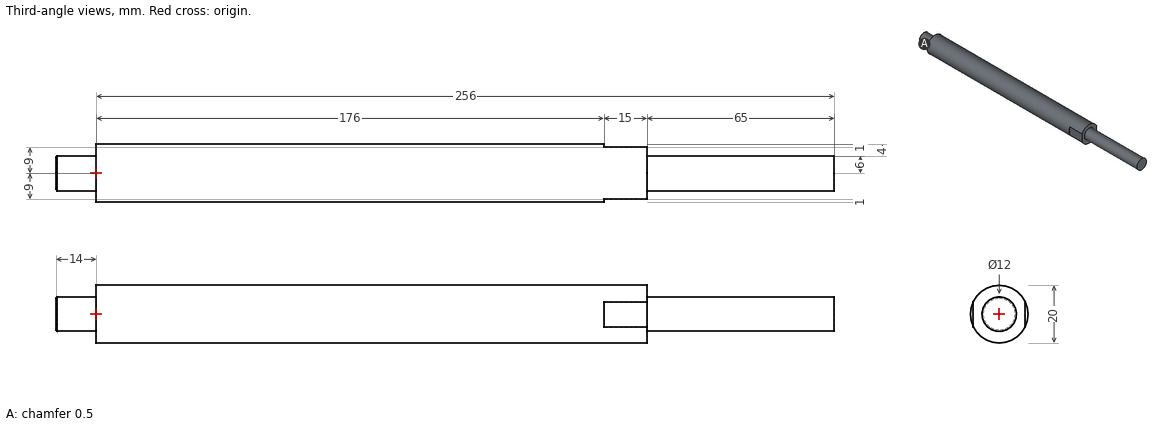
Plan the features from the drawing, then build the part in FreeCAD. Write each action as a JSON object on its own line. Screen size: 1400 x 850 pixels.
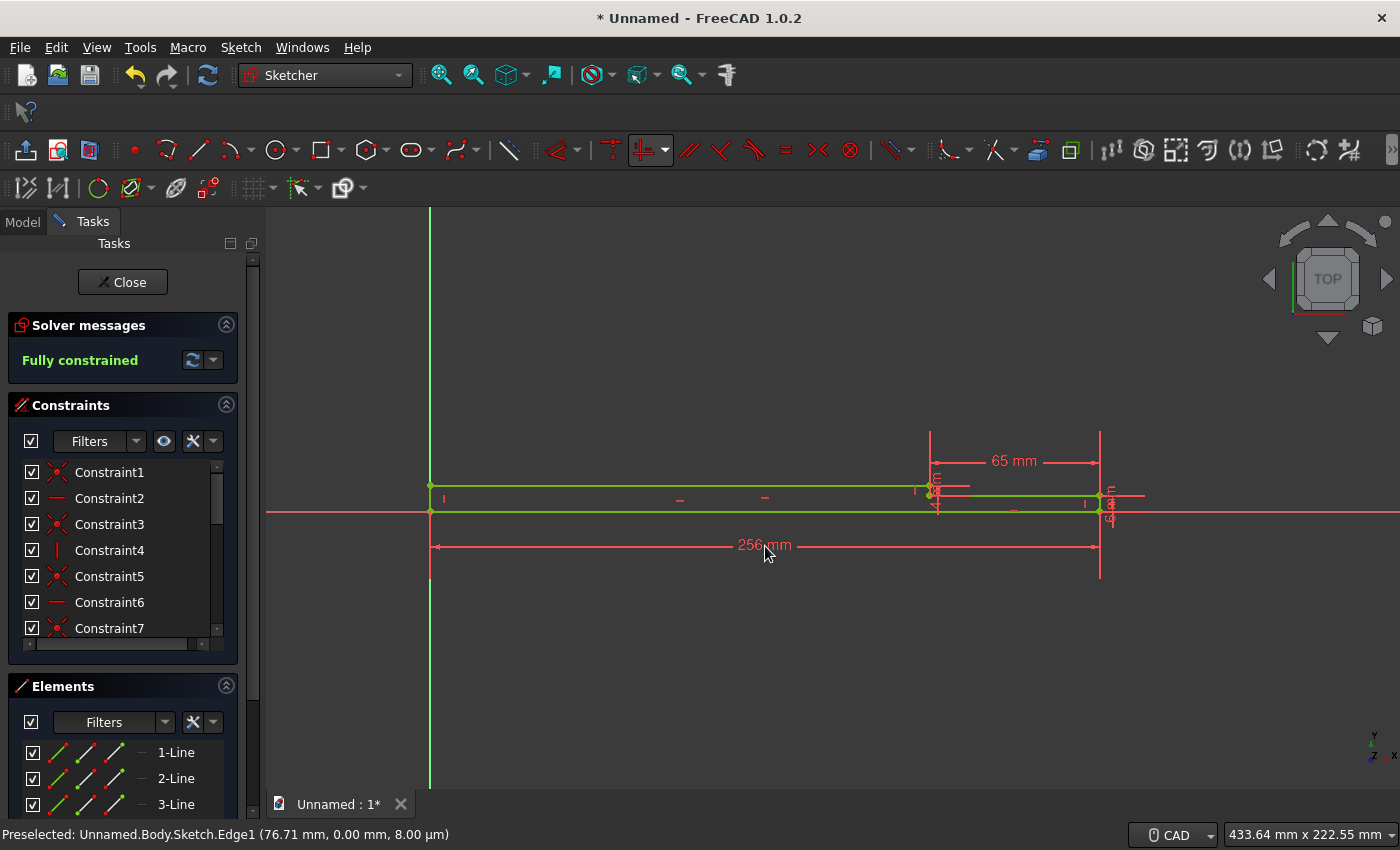
{"action": "left_click", "coordinate": [123, 282]}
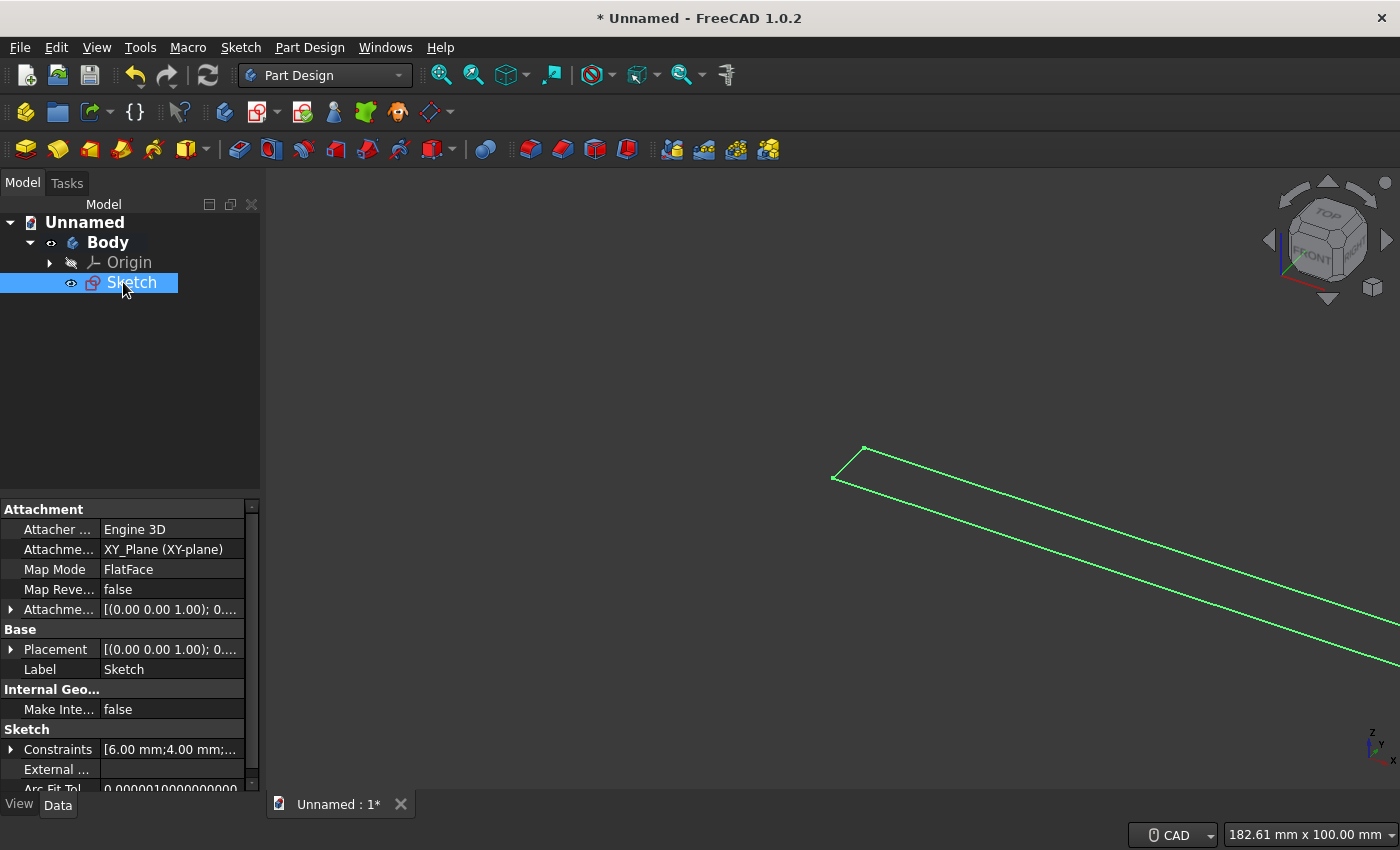
{"action": "left_click", "coordinate": [58, 150]}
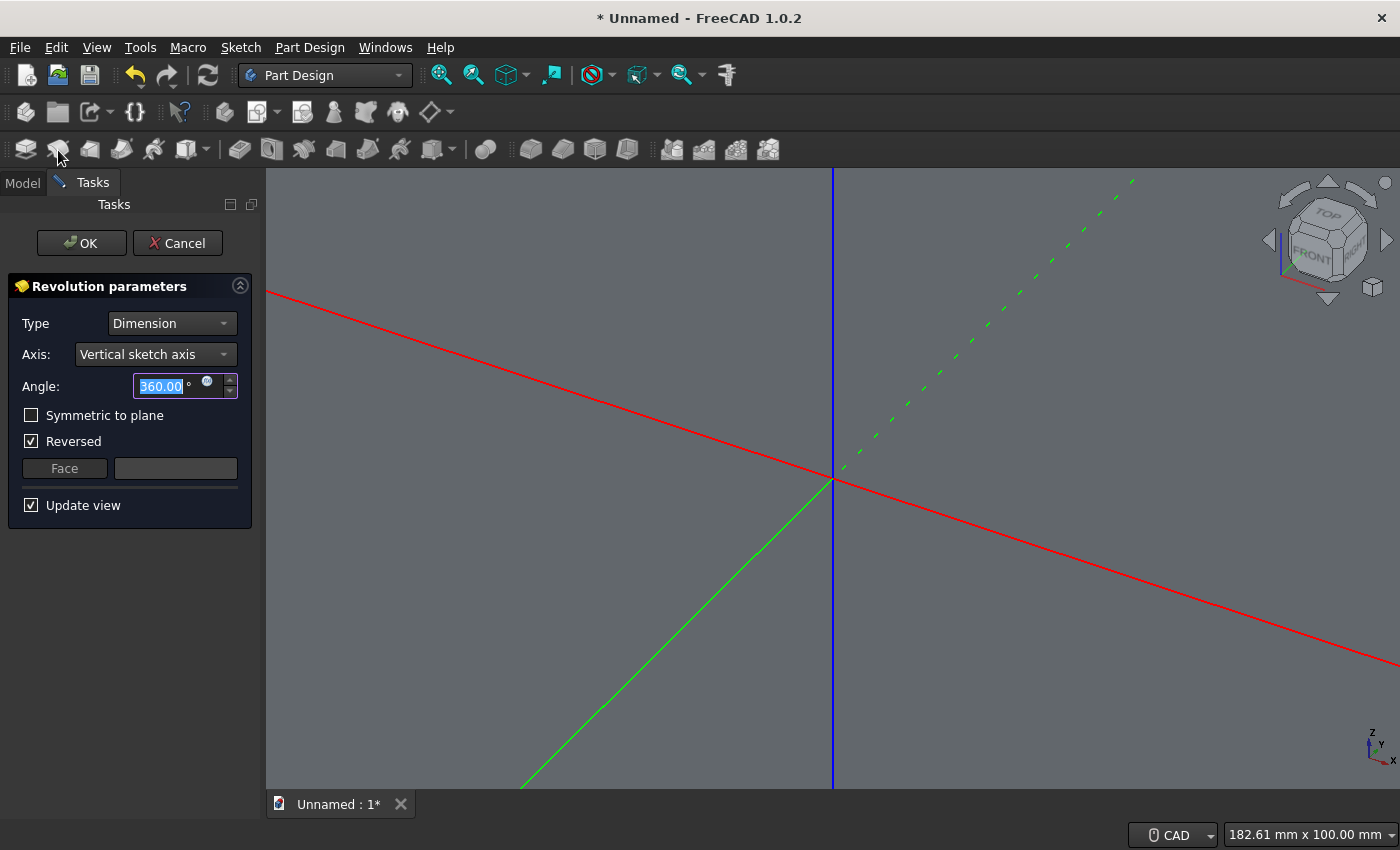
{"action": "left_click", "coordinate": [156, 354]}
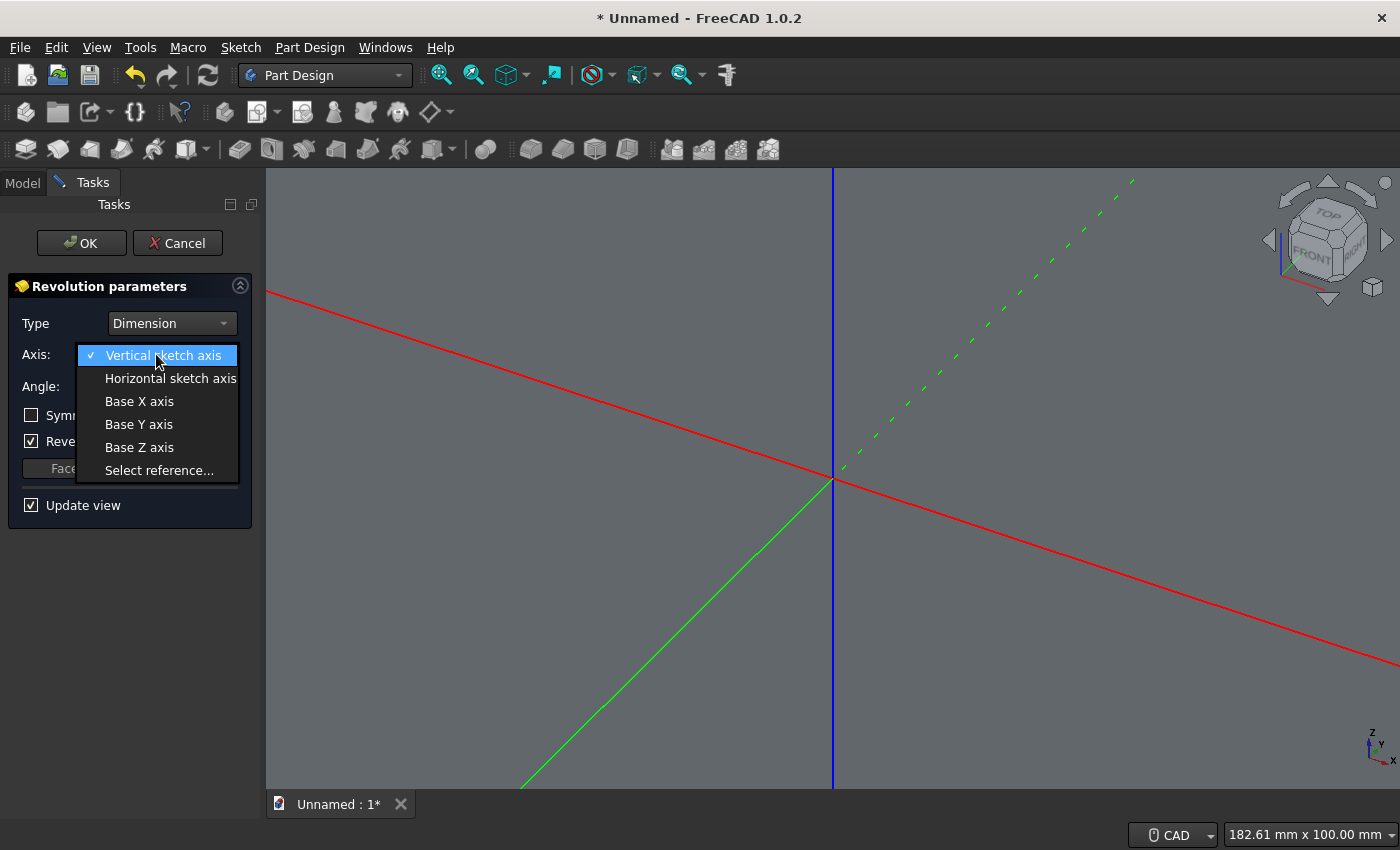
{"action": "left_click", "coordinate": [156, 378]}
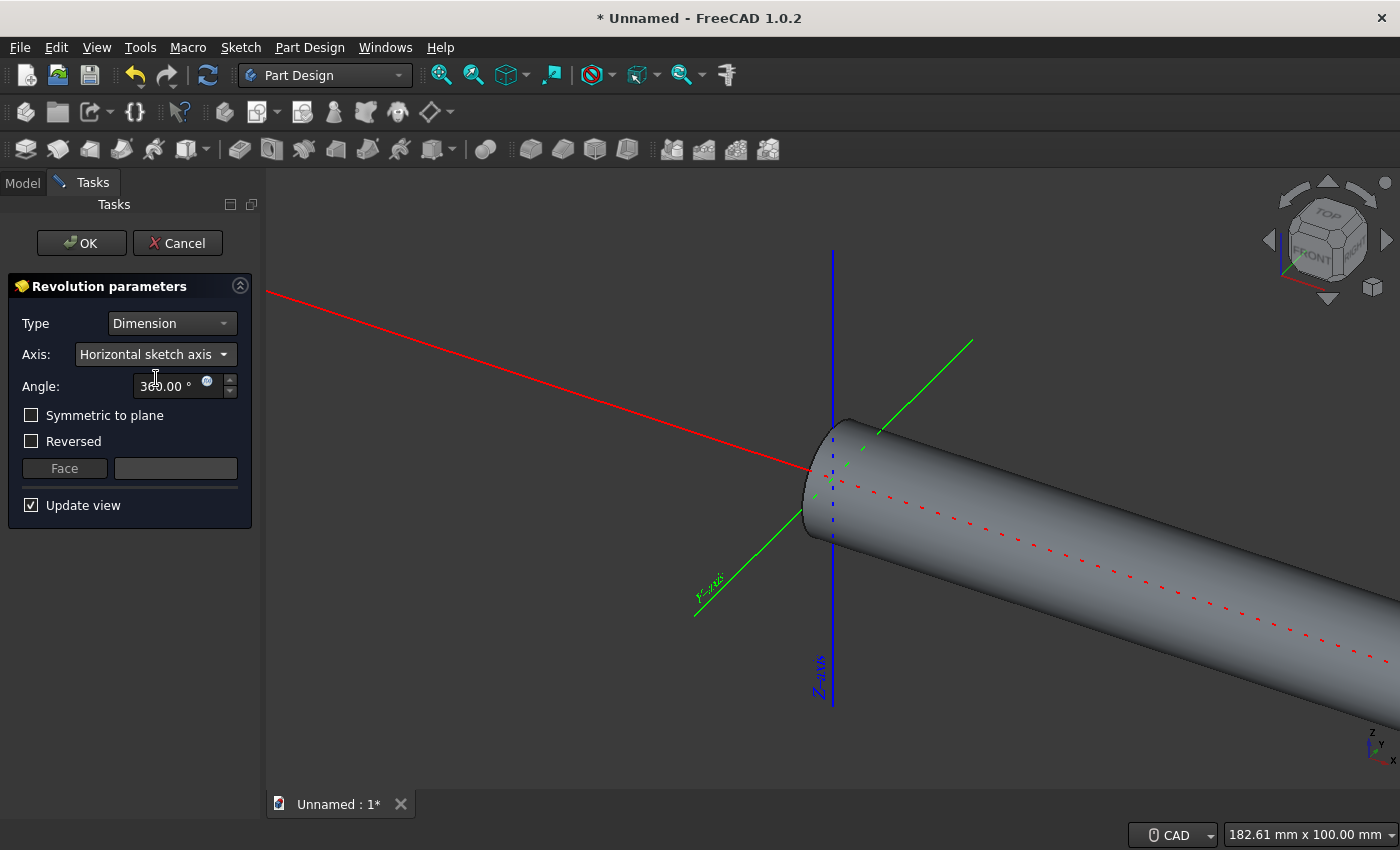
{"action": "left_click", "coordinate": [82, 243]}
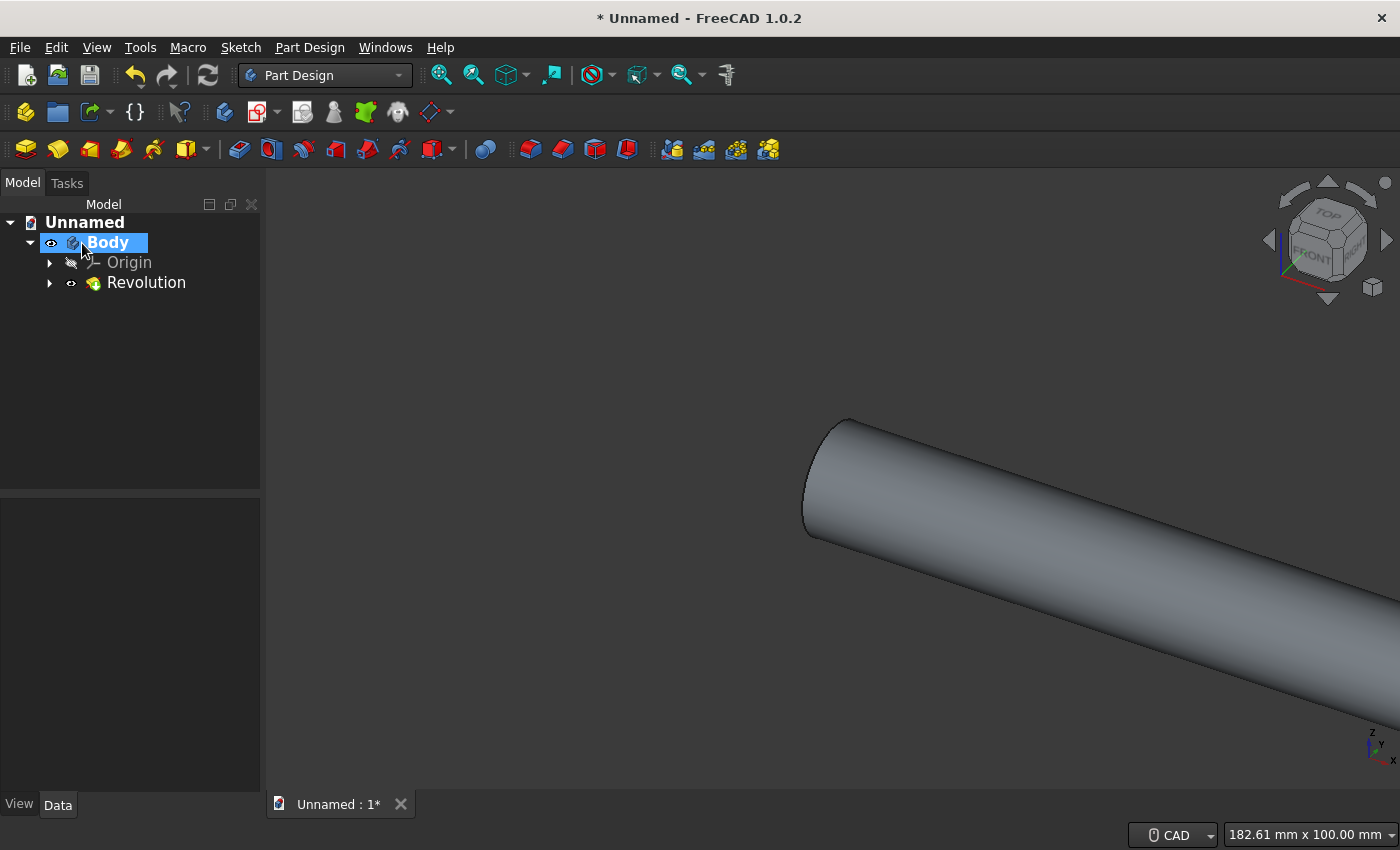
{"action": "key", "text": "v f"}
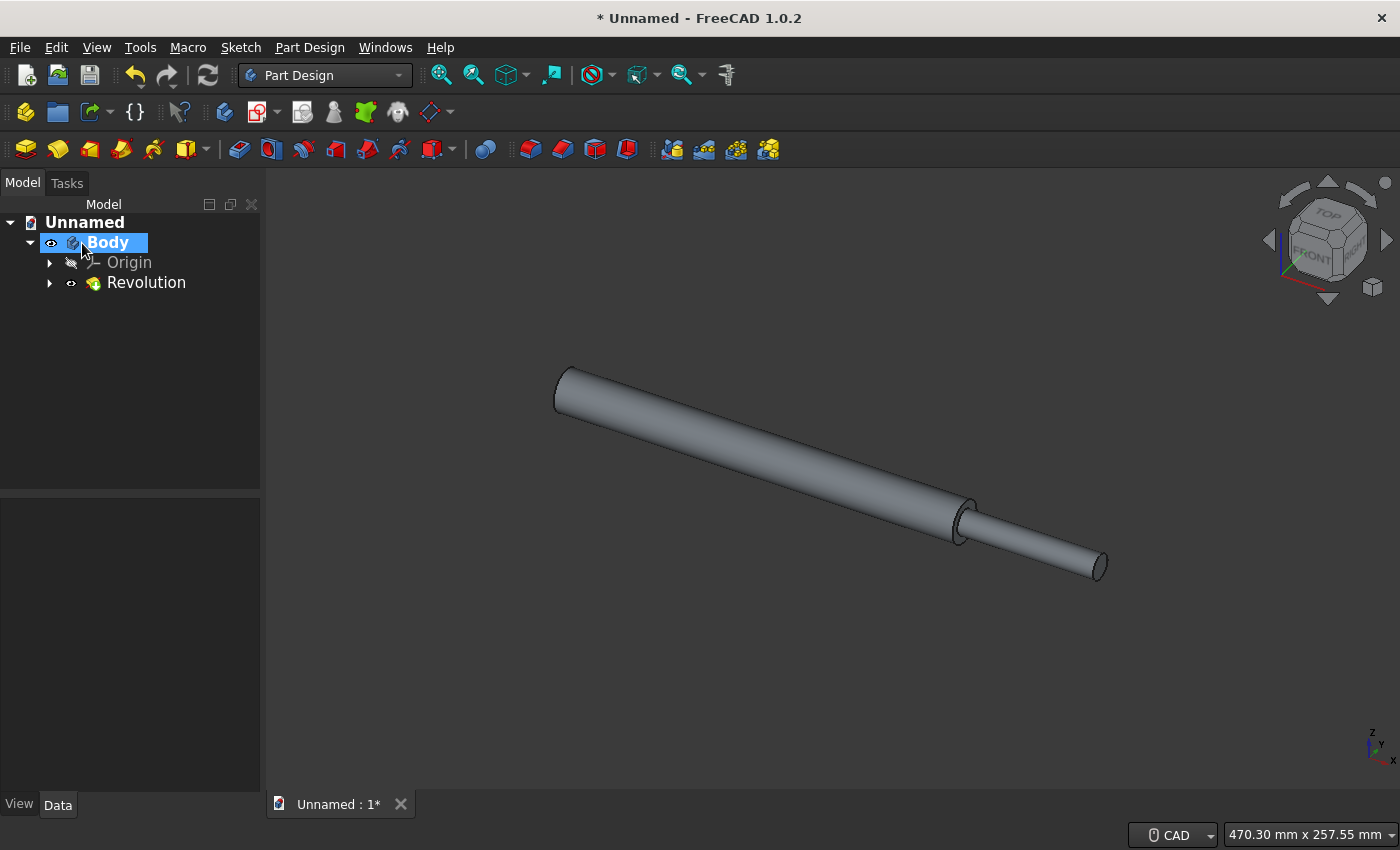
{"action": "left_click", "coordinate": [258, 112]}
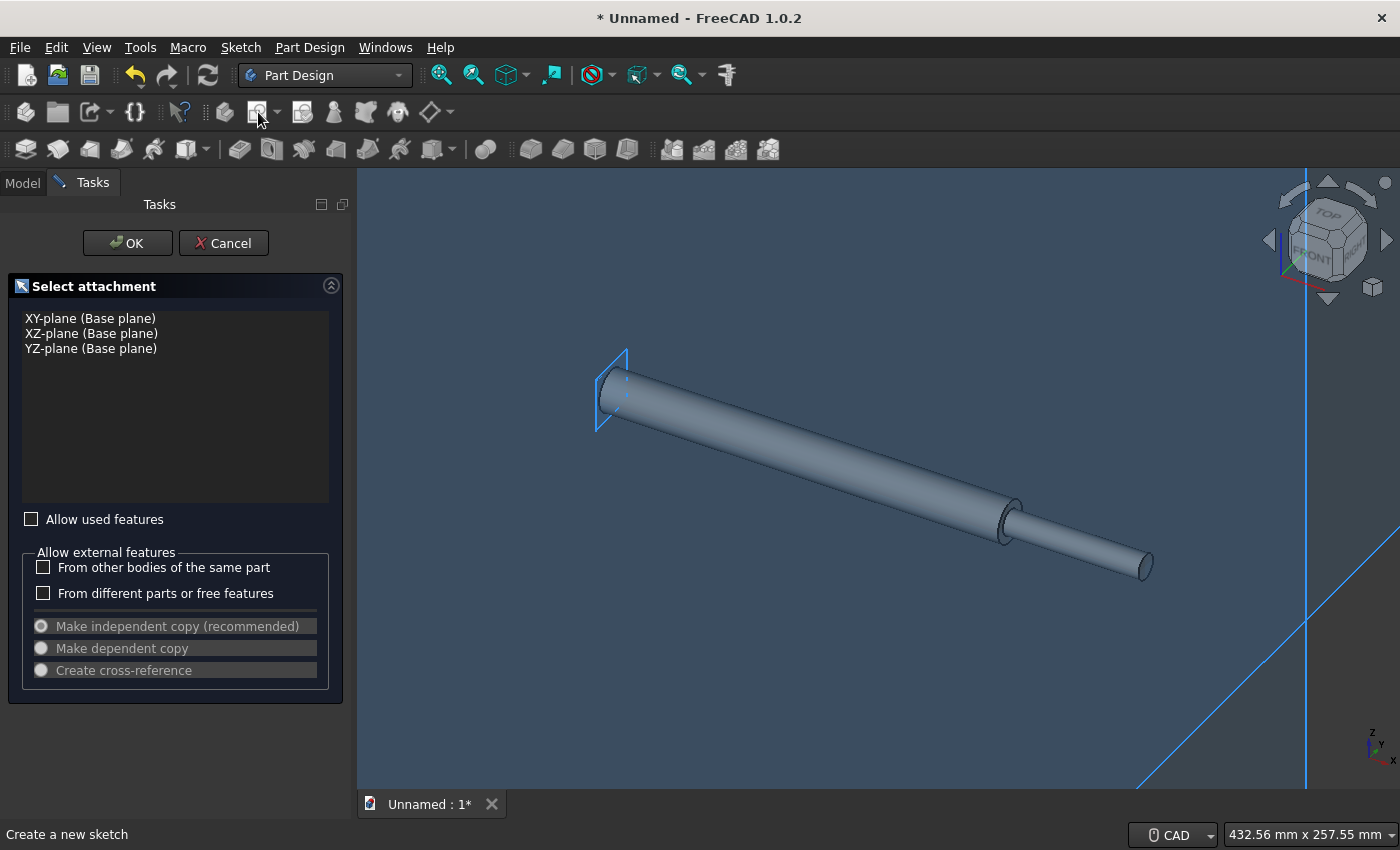
{"action": "left_click", "coordinate": [82, 348]}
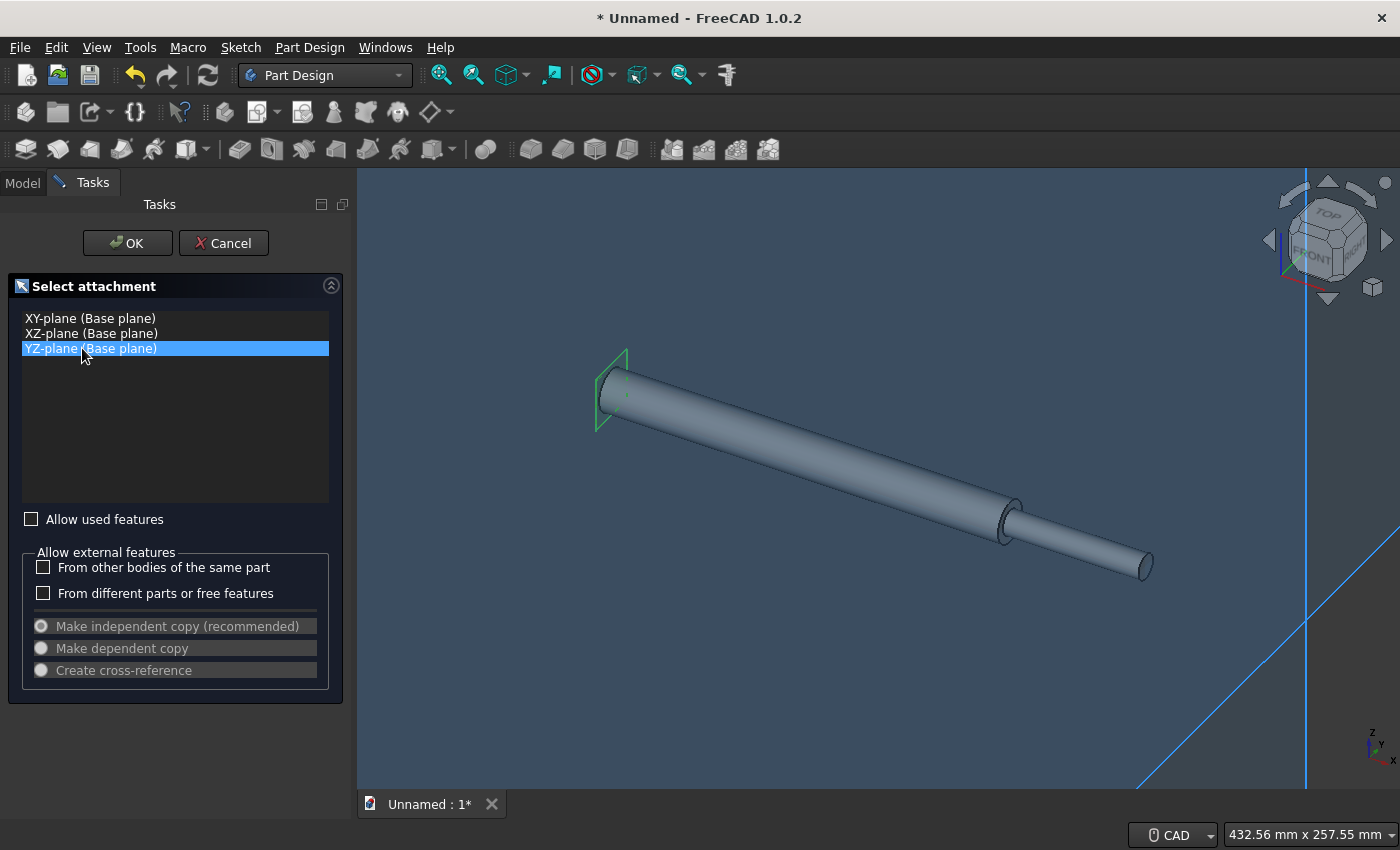
{"action": "left_click", "coordinate": [128, 243]}